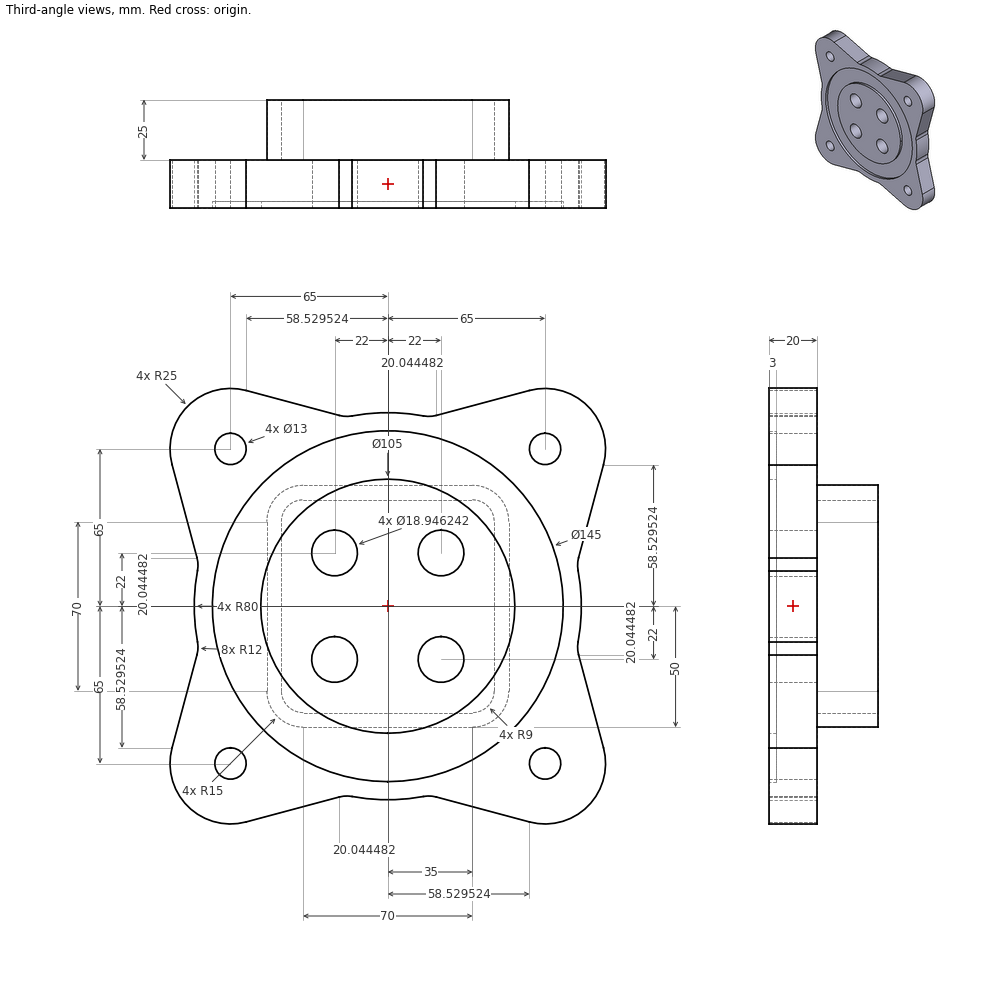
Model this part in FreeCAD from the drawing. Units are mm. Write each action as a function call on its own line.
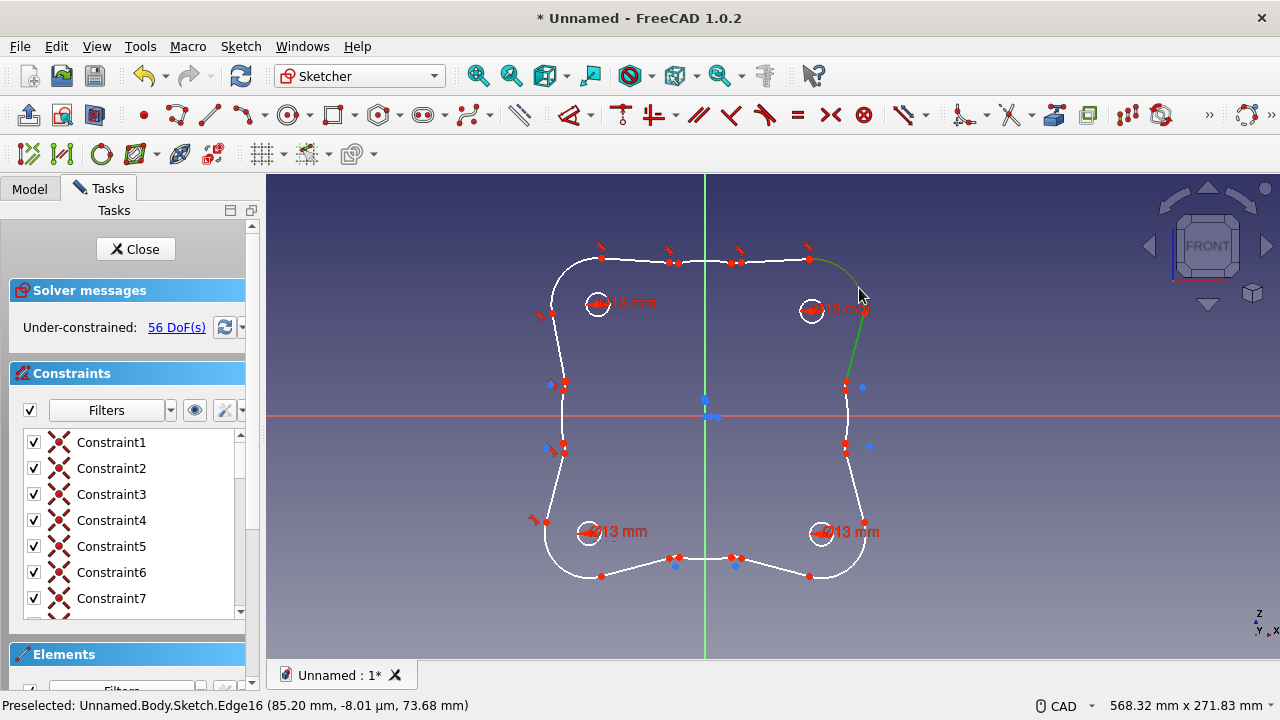
click(765, 116)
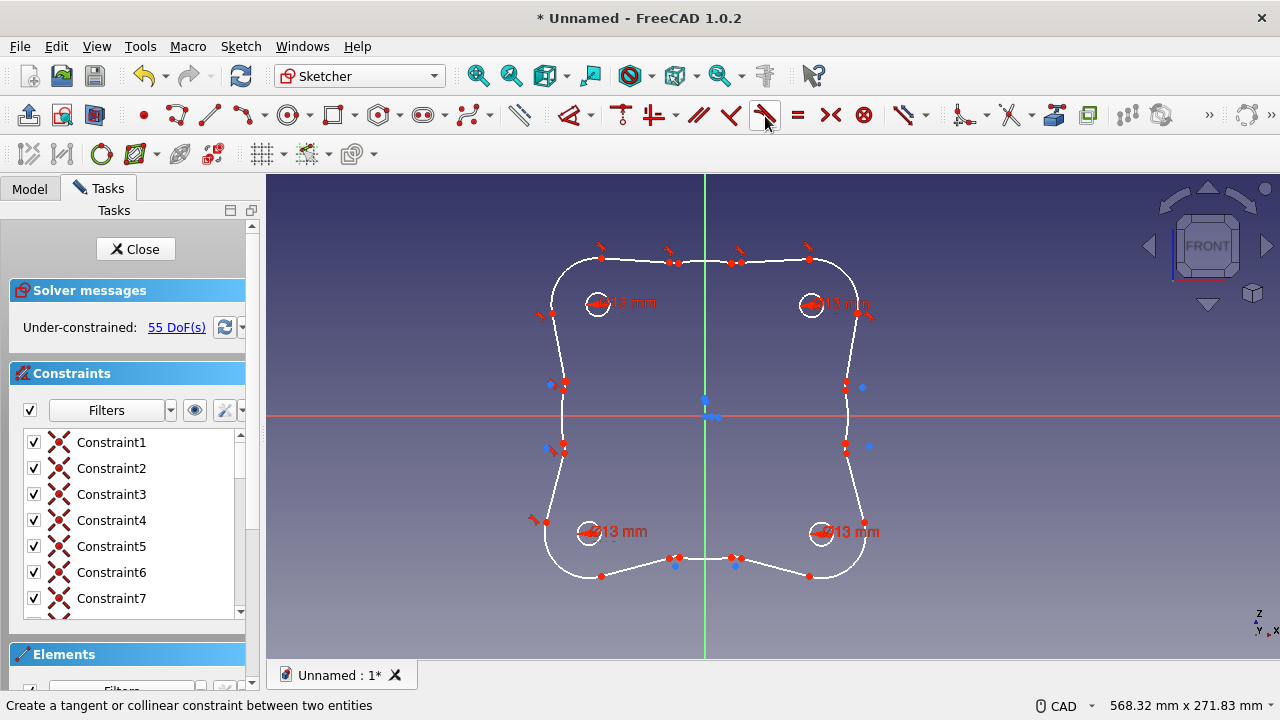
click(854, 334)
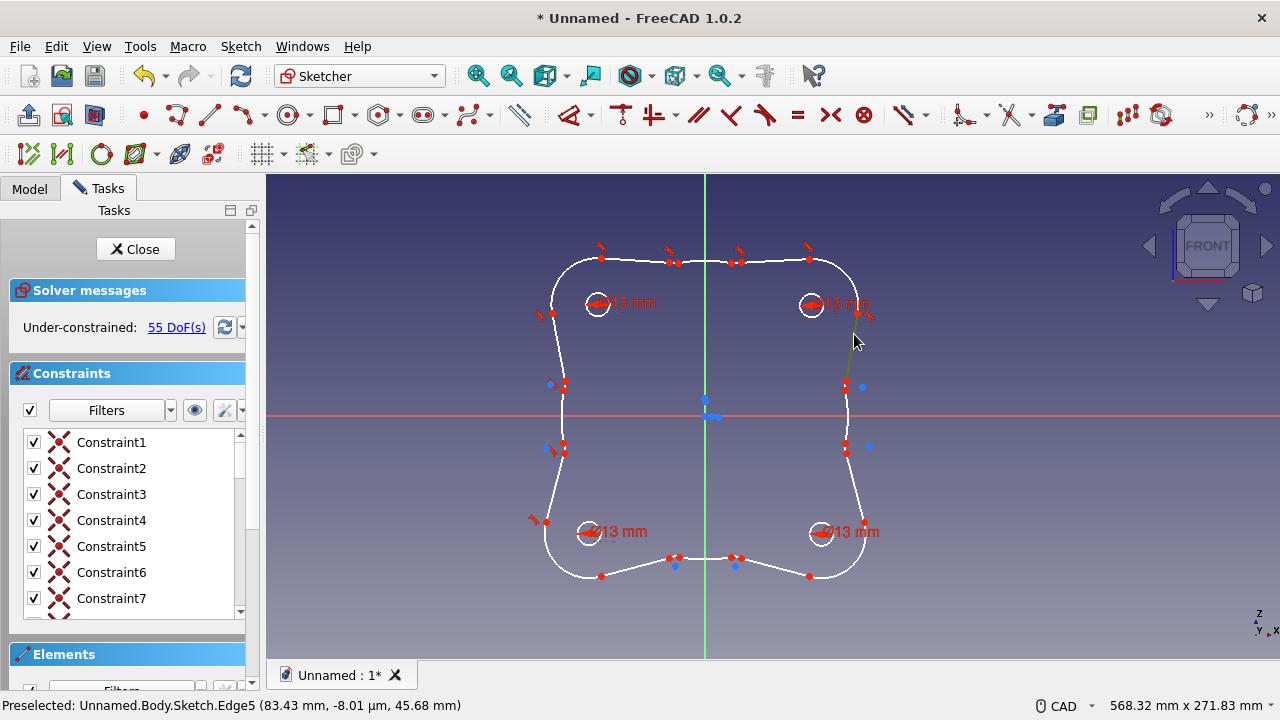
scroll(845, 386, up, 6)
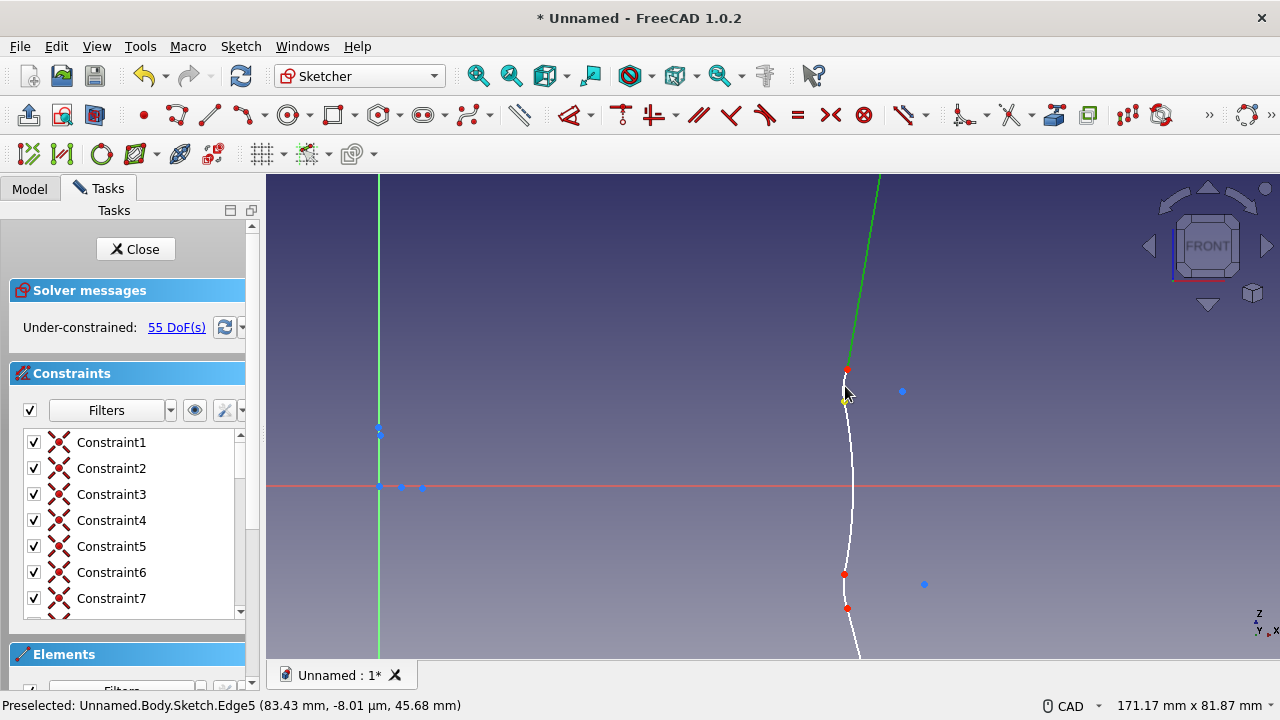
click(844, 385)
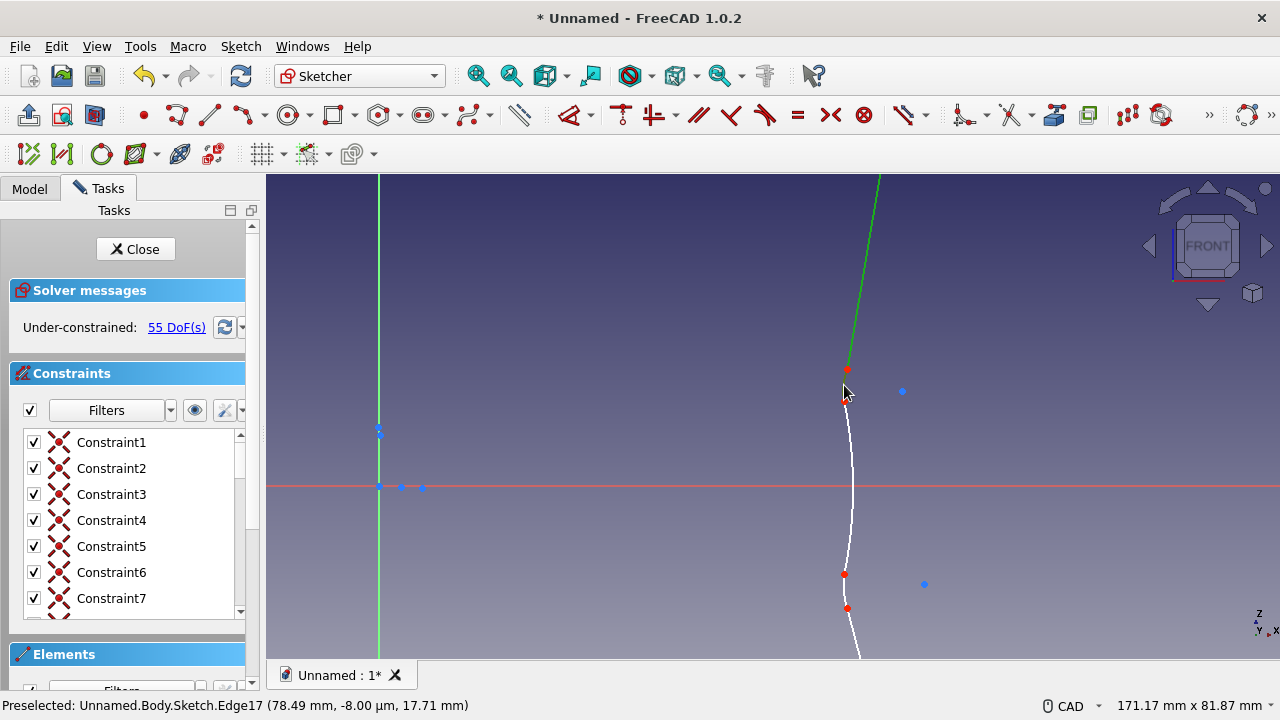
click(765, 116)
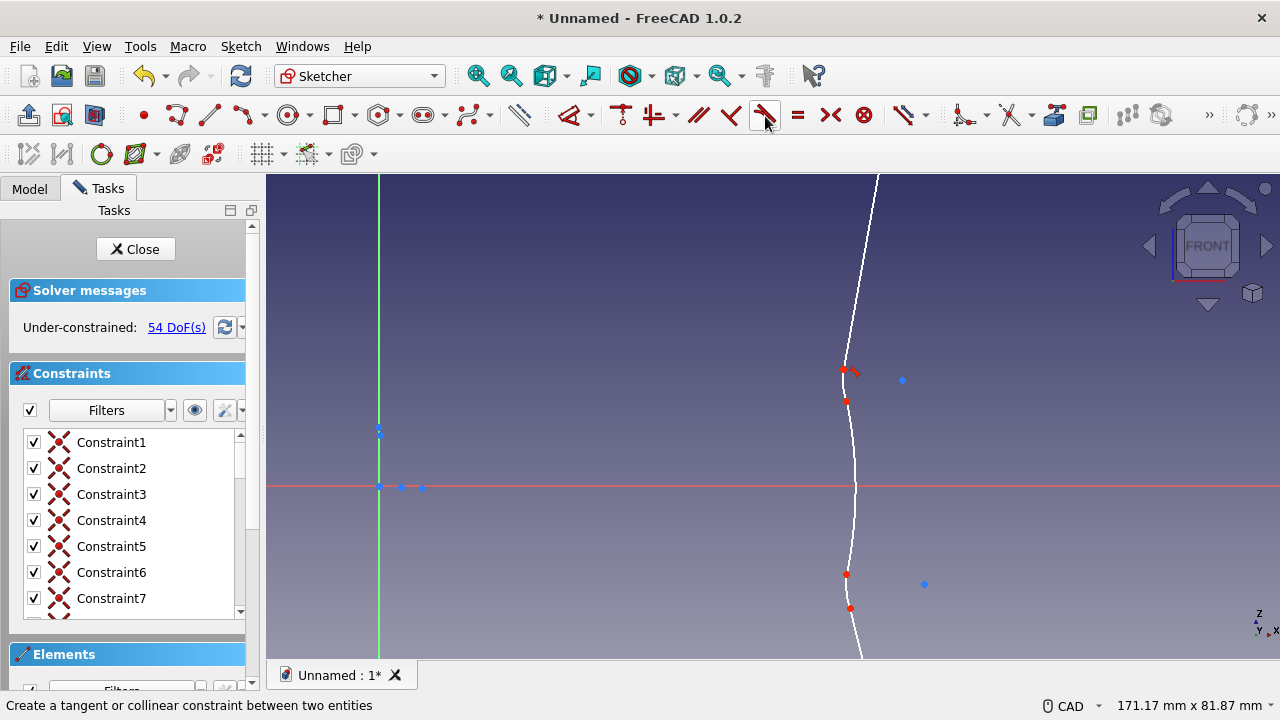
scroll(845, 386, down, 6)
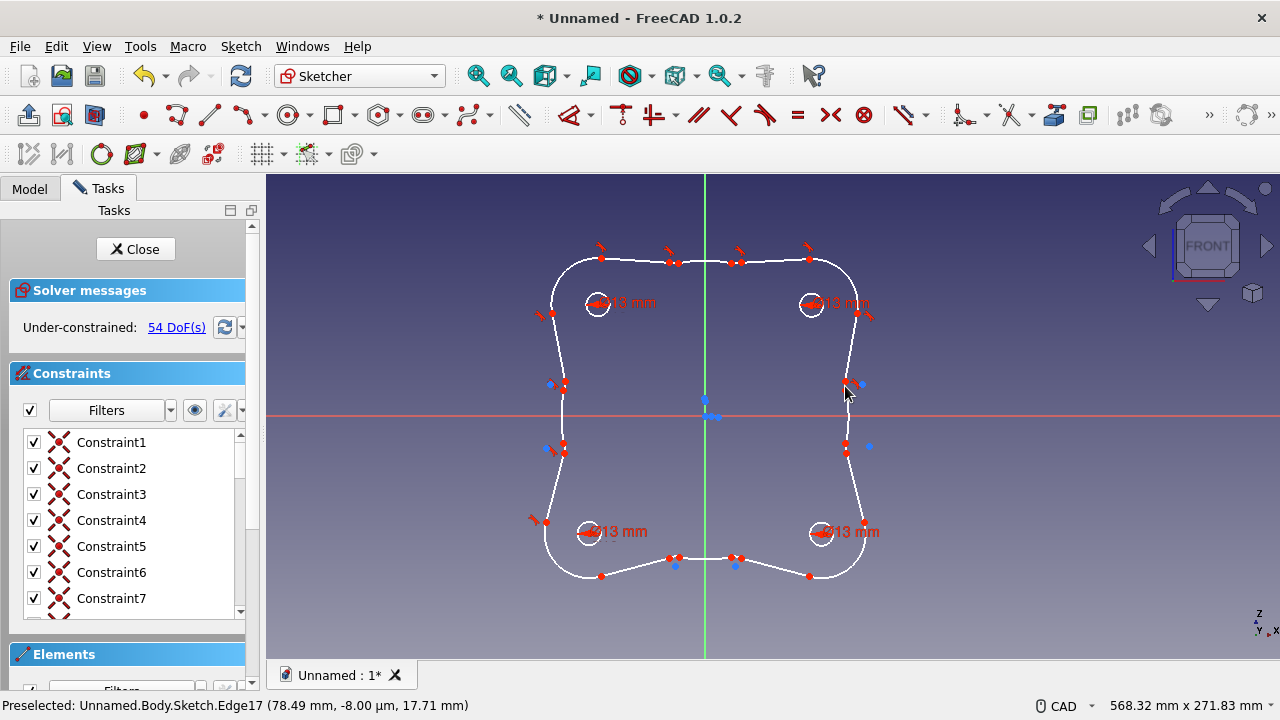
click(852, 474)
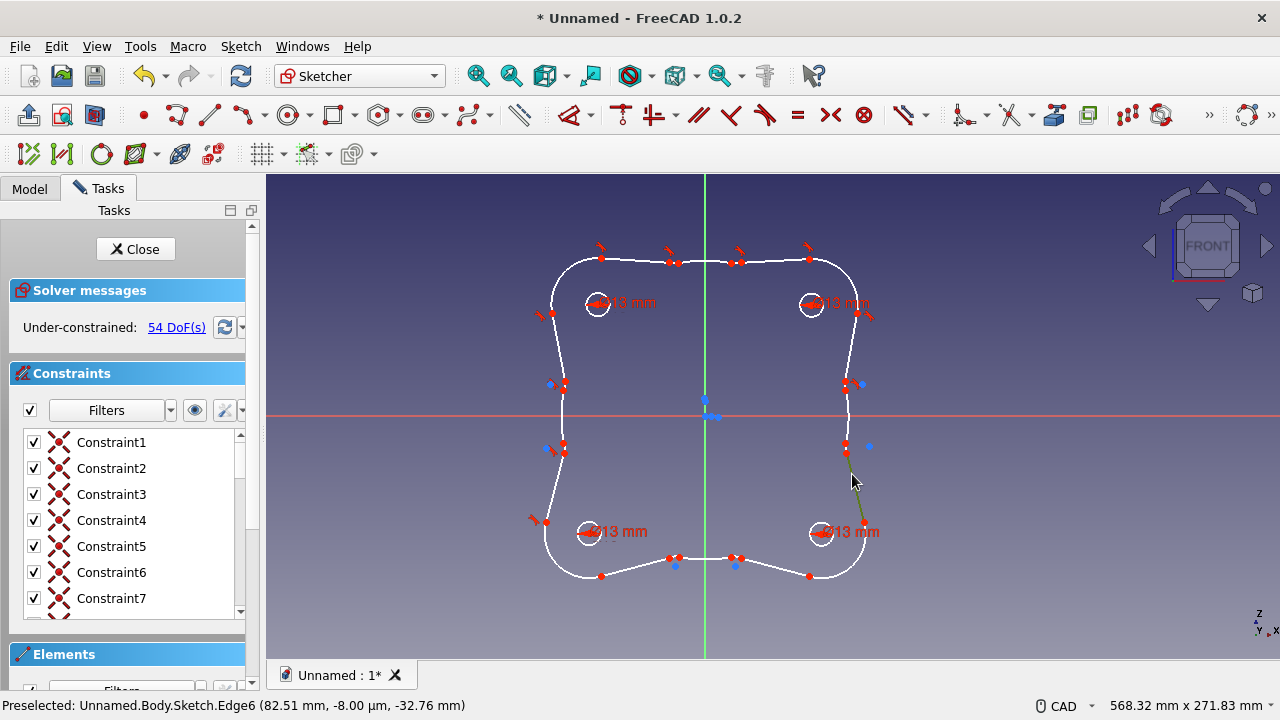
scroll(846, 448, up, 5)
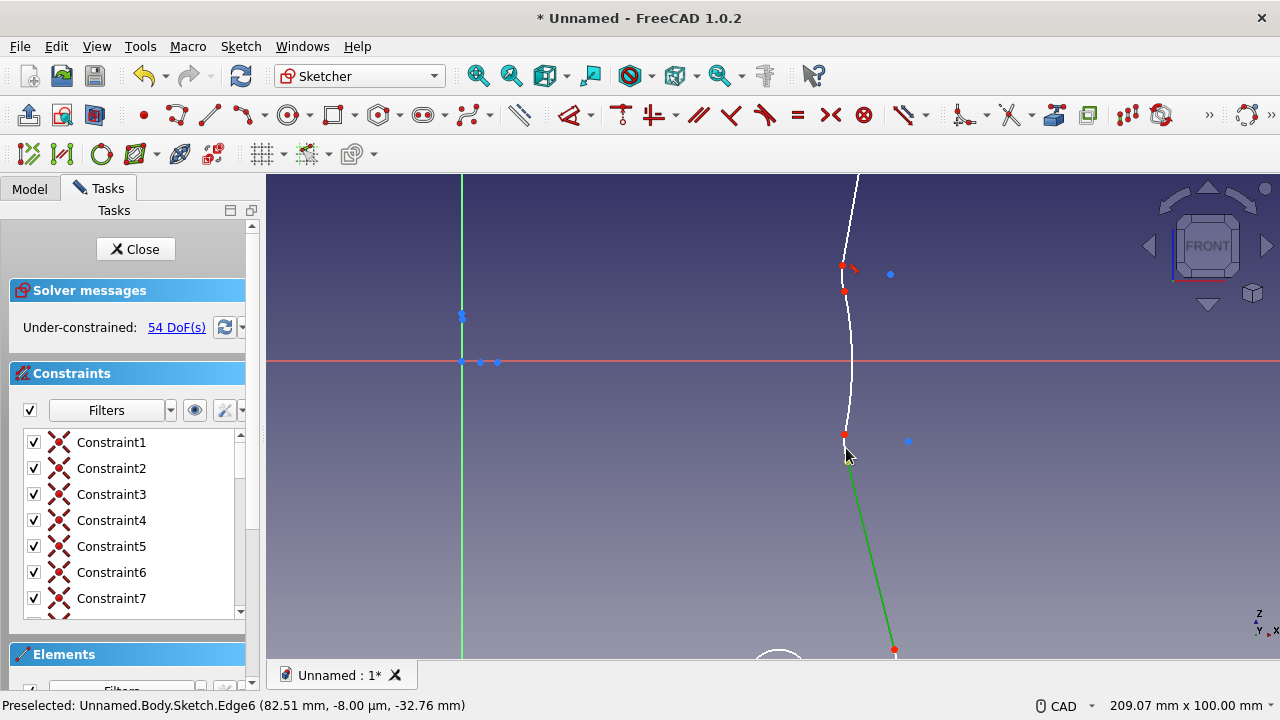
click(845, 448)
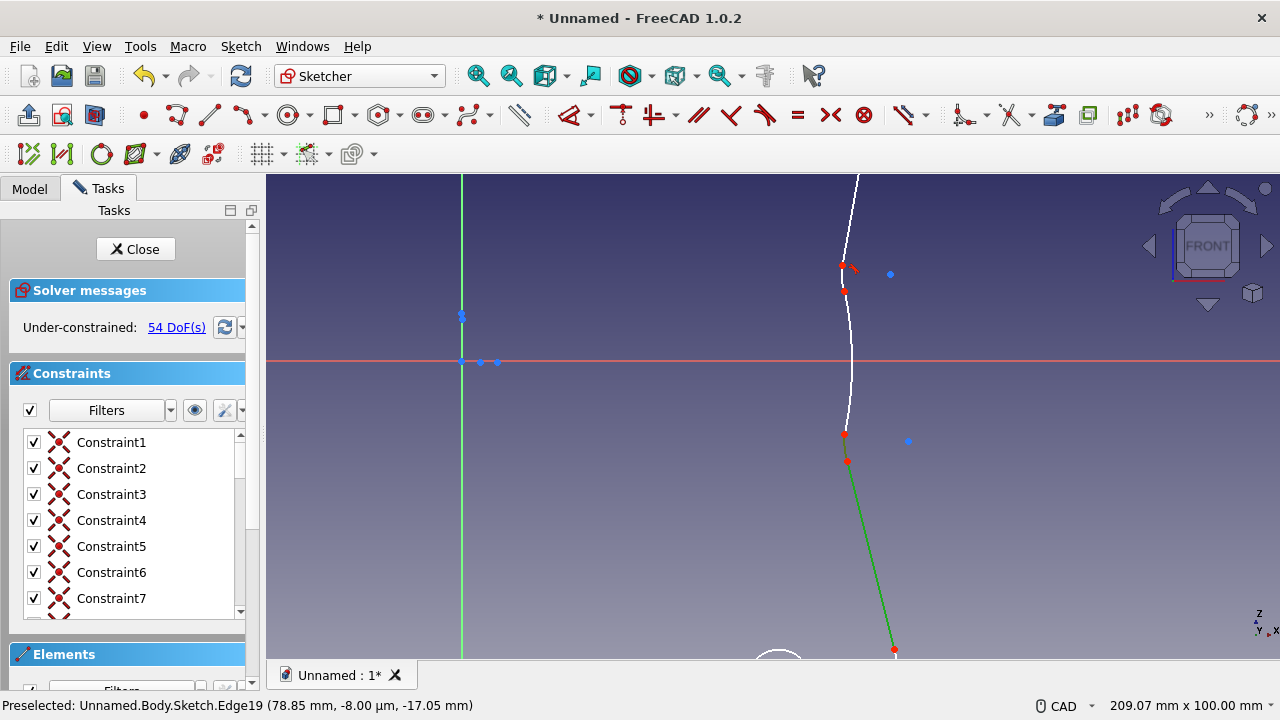
click(765, 116)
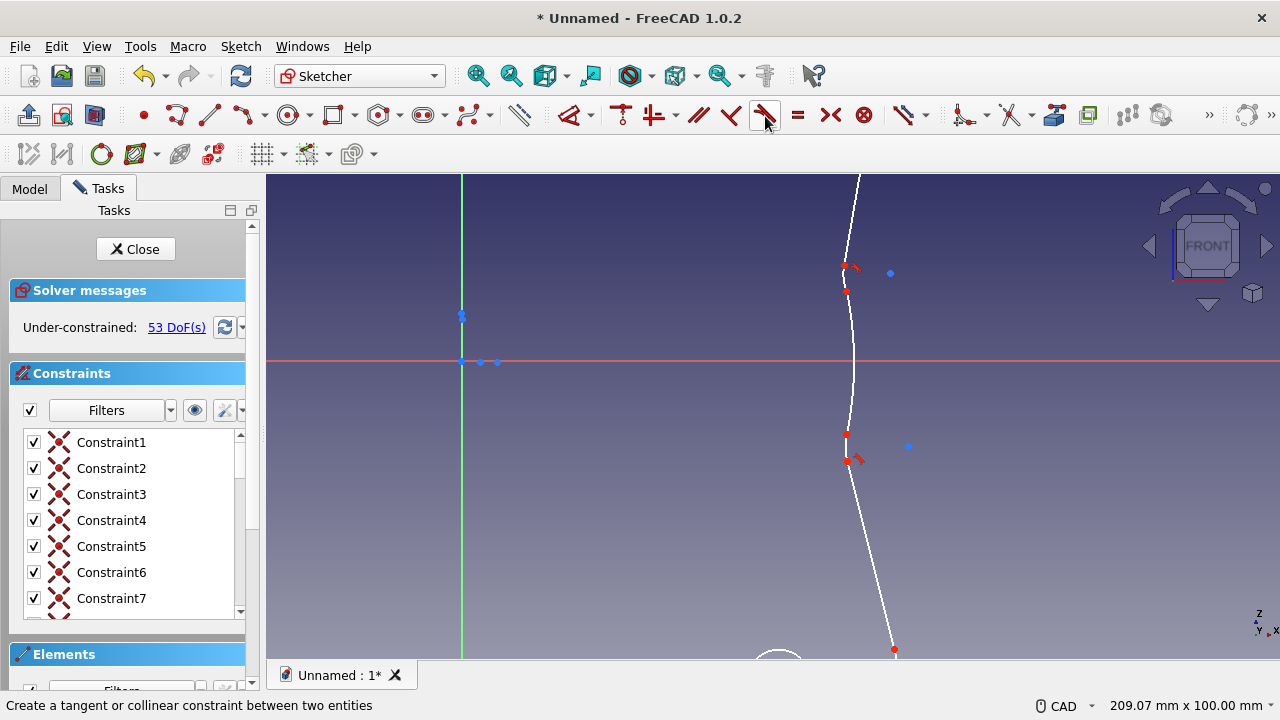
click(862, 518)